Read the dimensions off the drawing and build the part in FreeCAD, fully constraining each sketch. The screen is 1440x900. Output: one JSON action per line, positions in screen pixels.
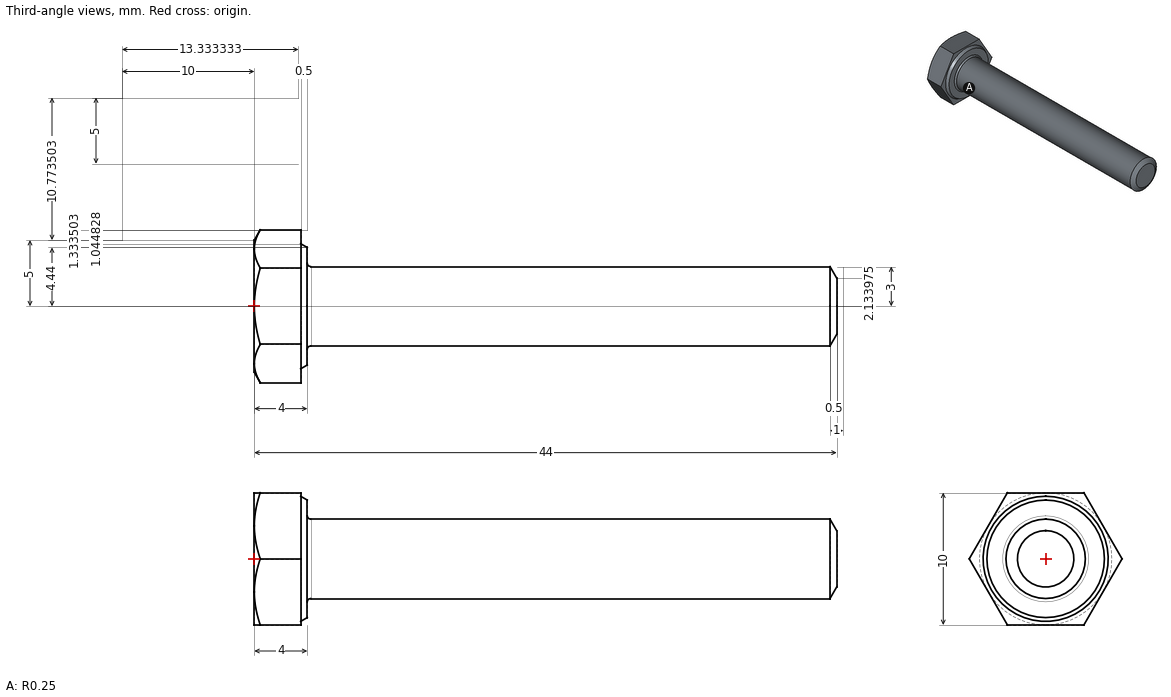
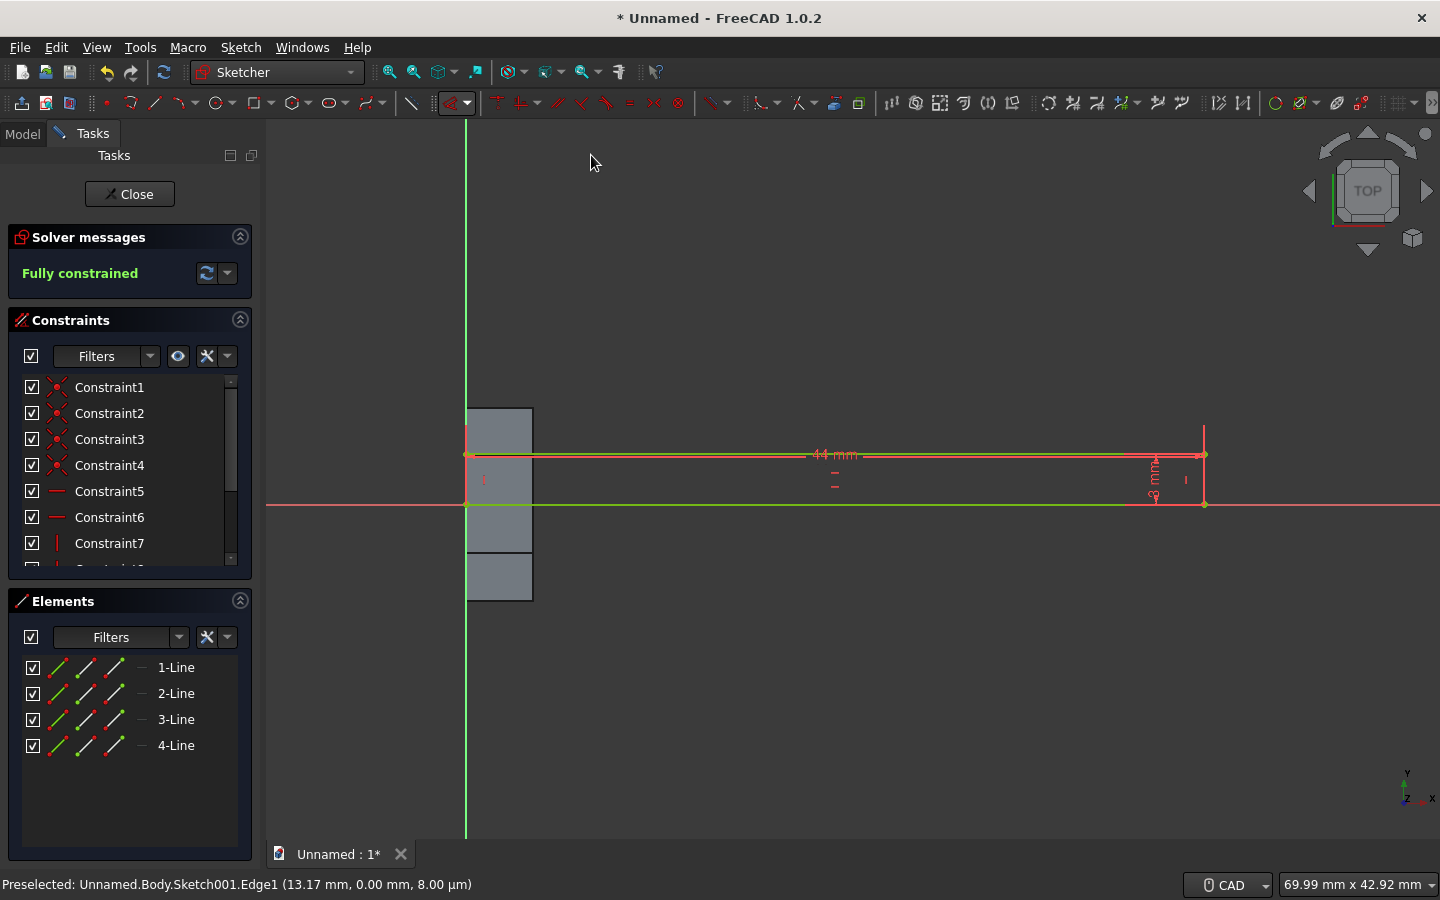
{"action": "left_click", "coordinate": [130, 194]}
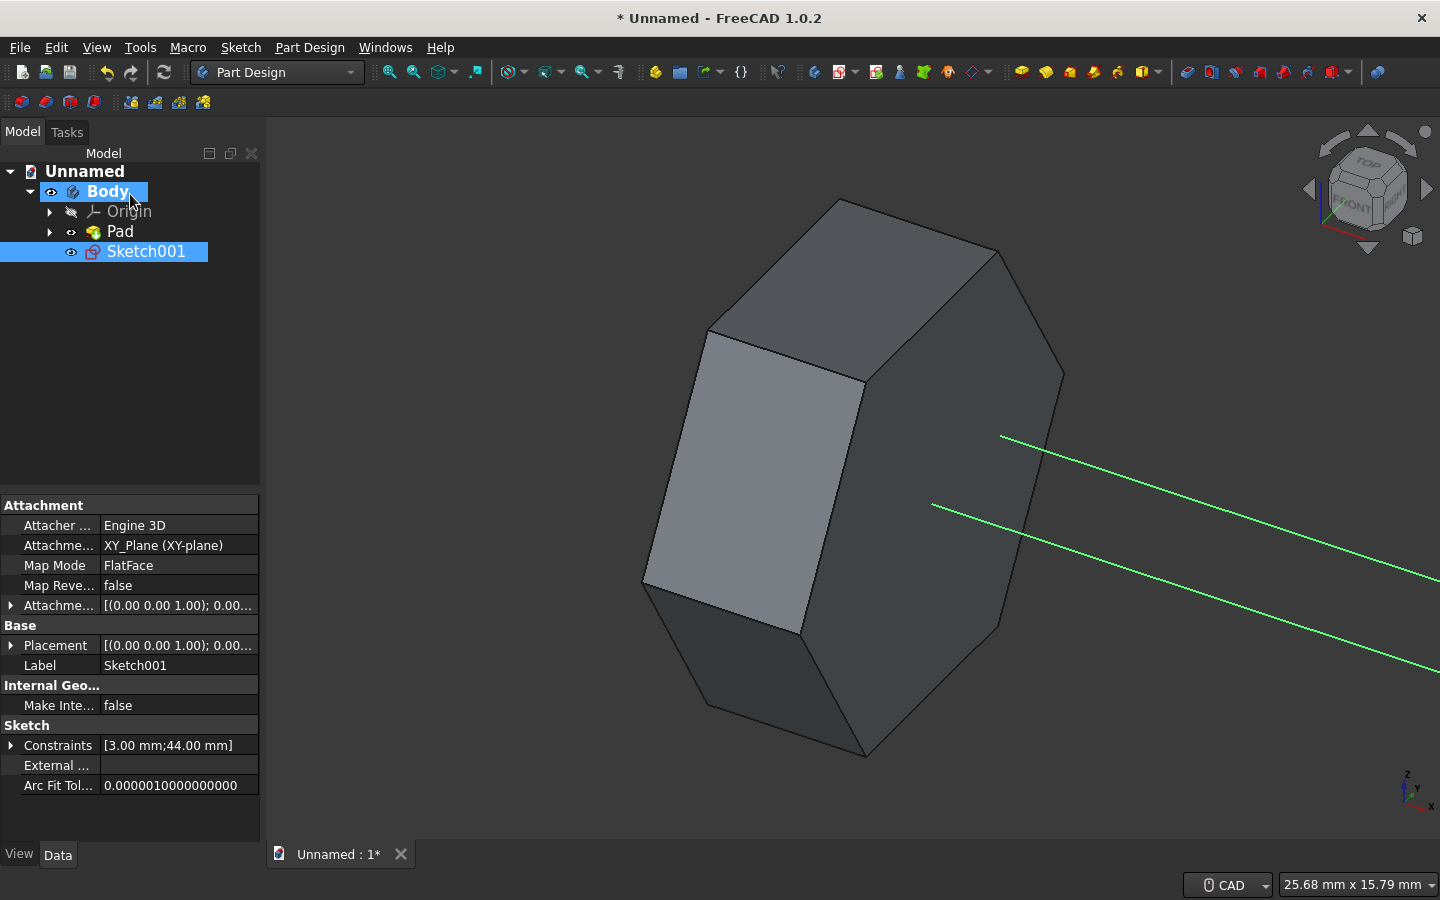
{"action": "left_click", "coordinate": [1046, 72]}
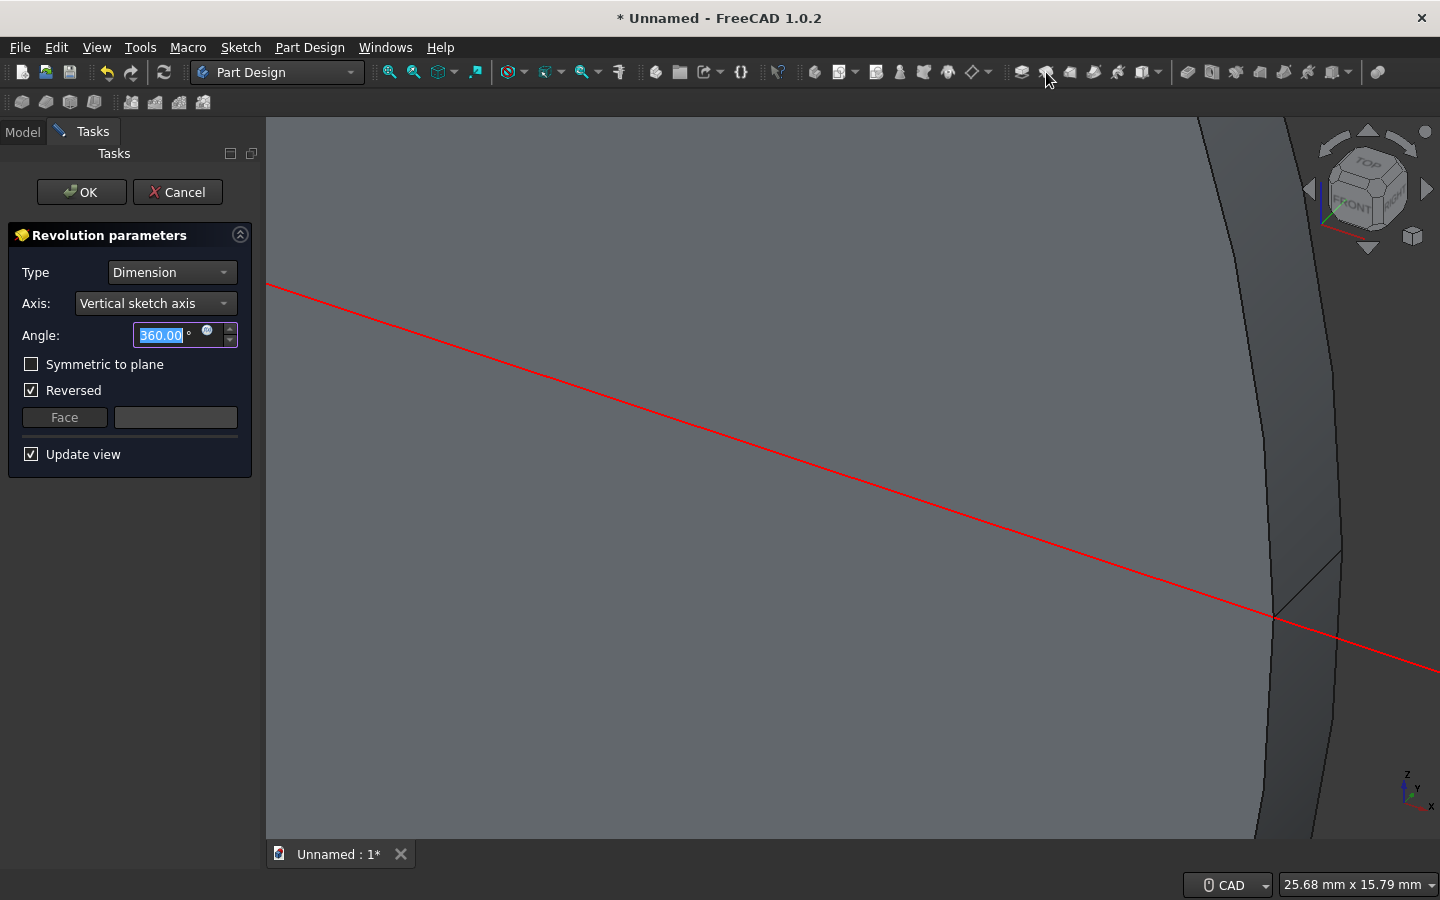
{"action": "left_click", "coordinate": [156, 304]}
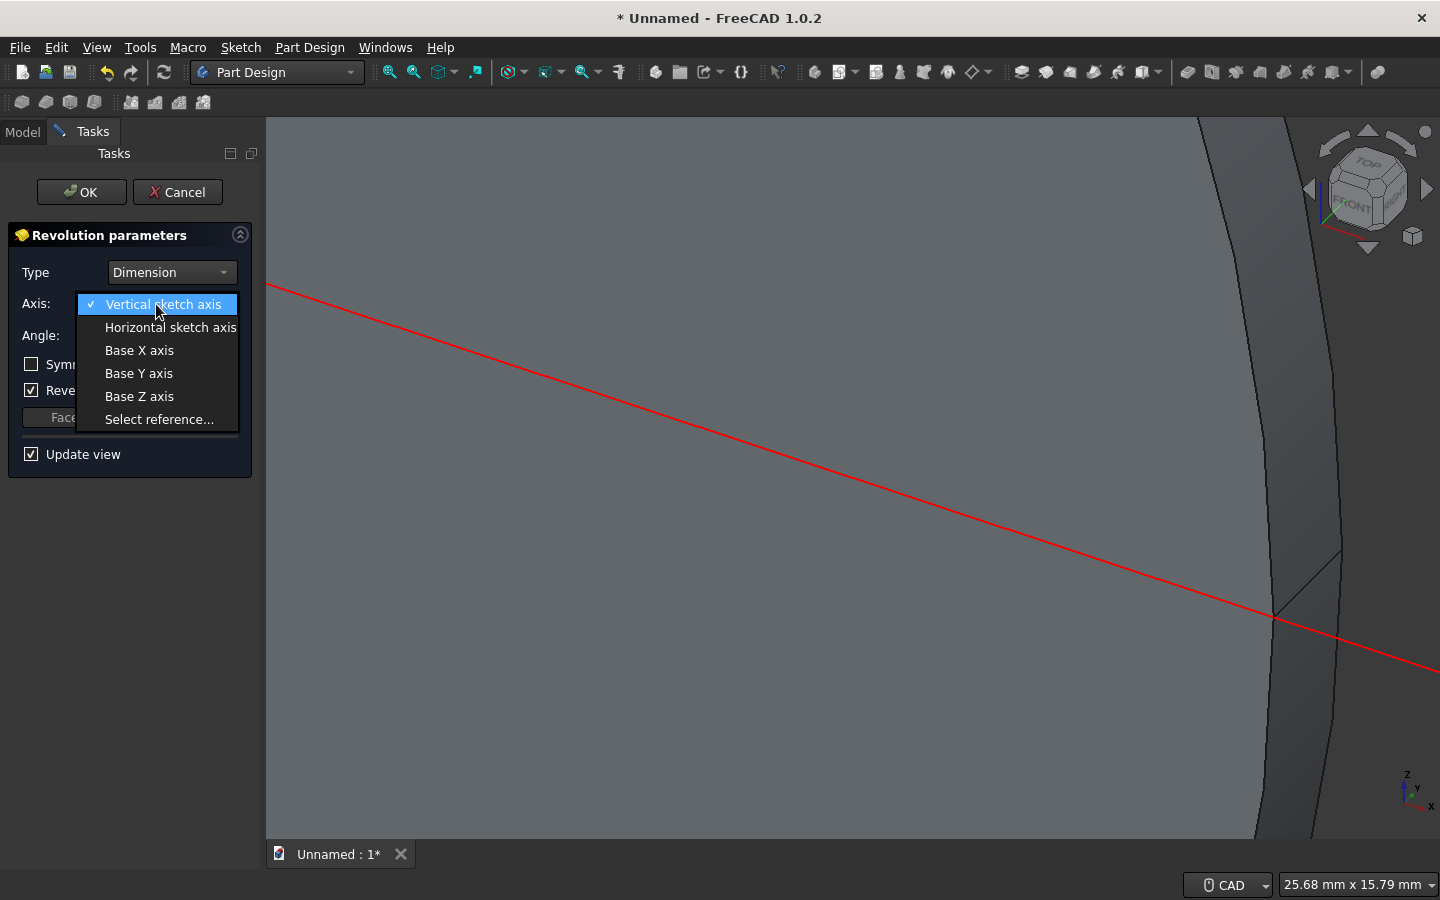
{"action": "left_click", "coordinate": [156, 328]}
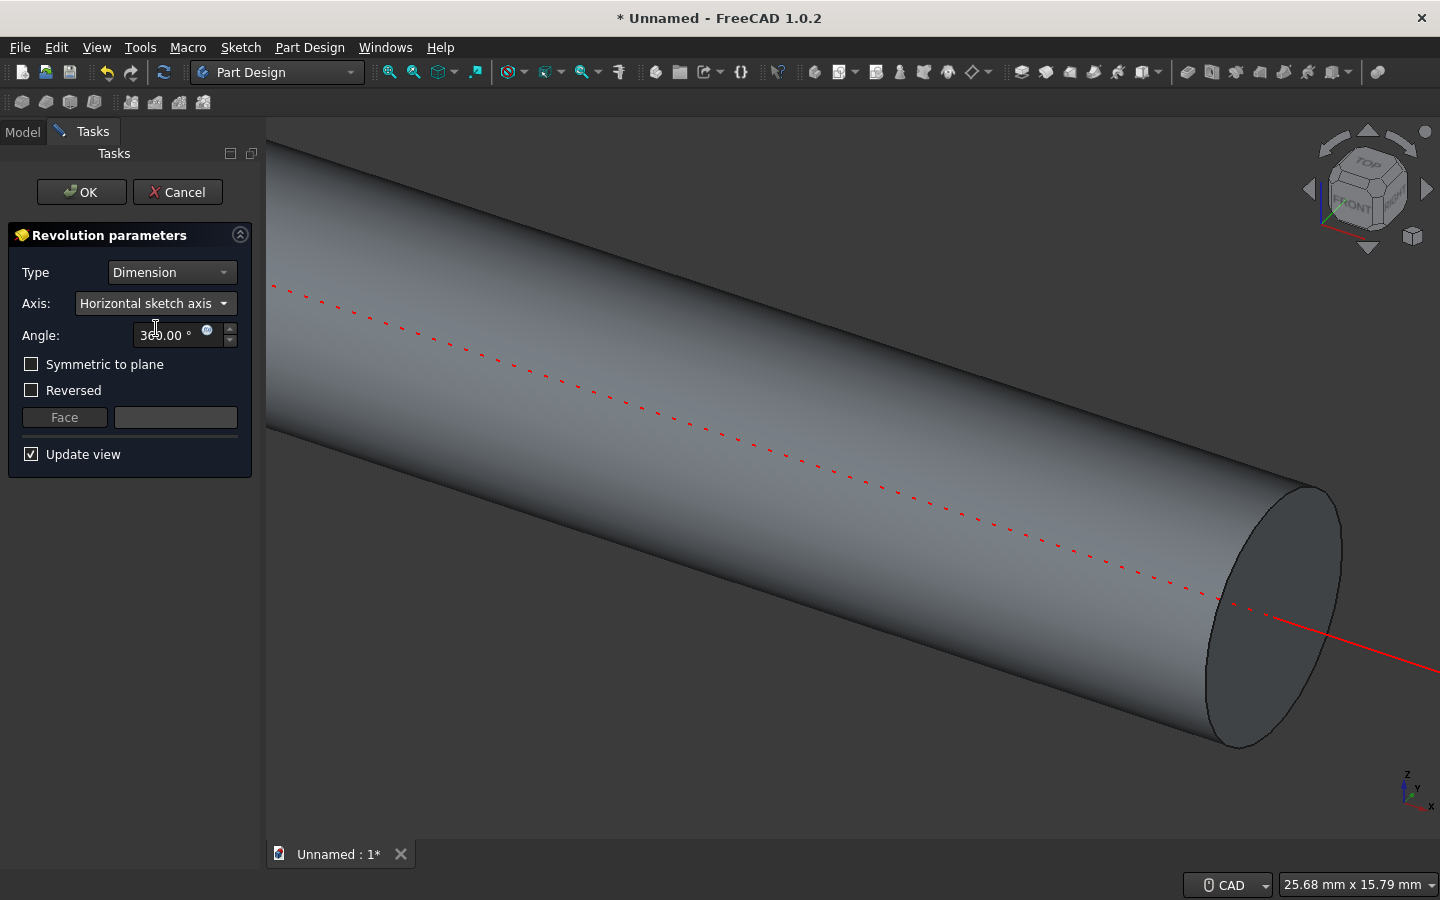
{"action": "left_click", "coordinate": [82, 192]}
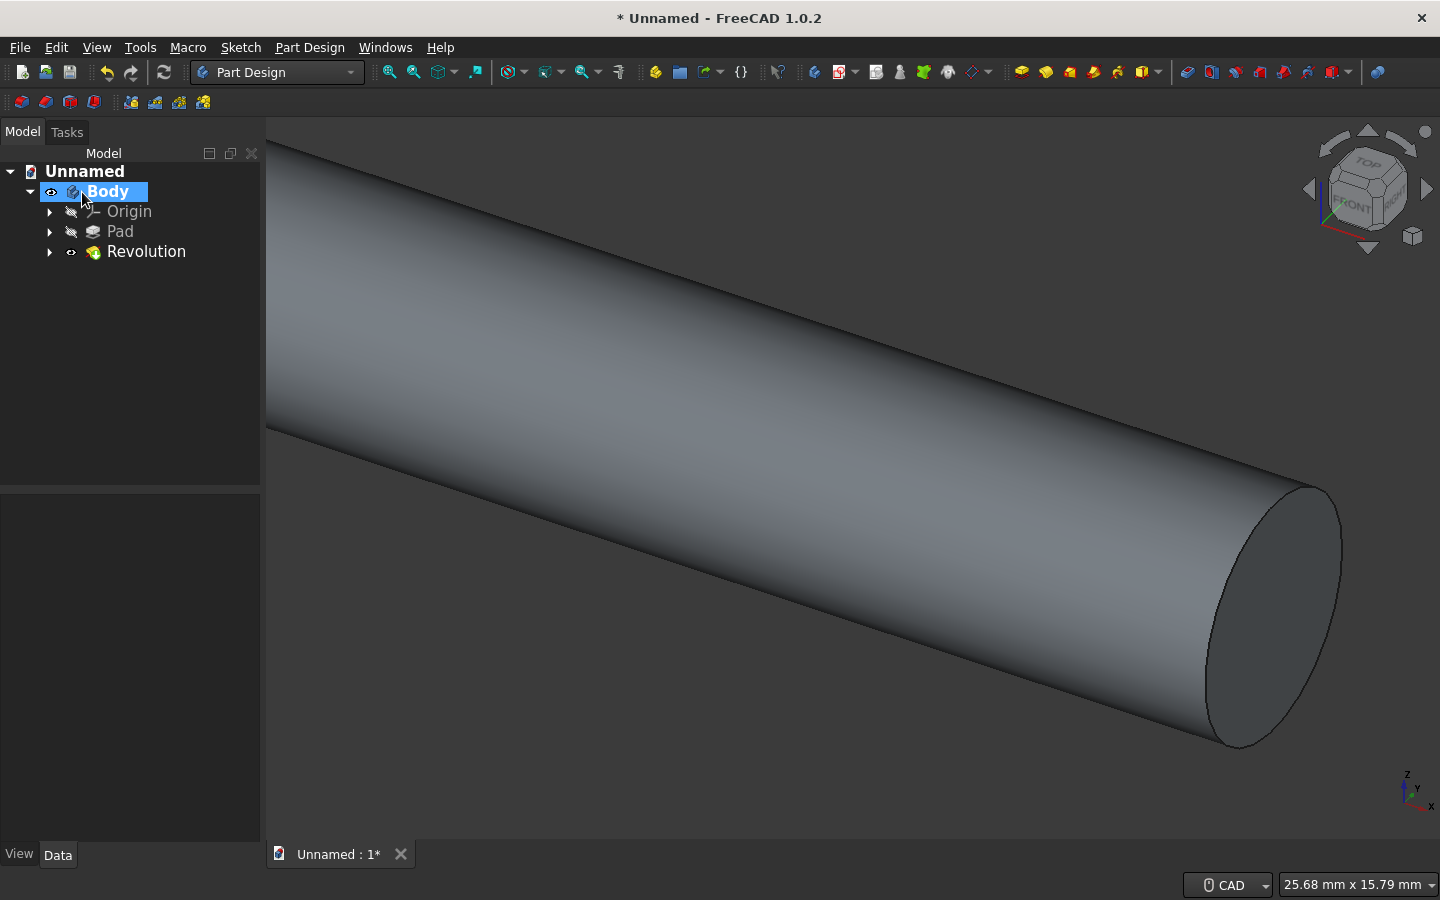
{"action": "left_click", "coordinate": [390, 72]}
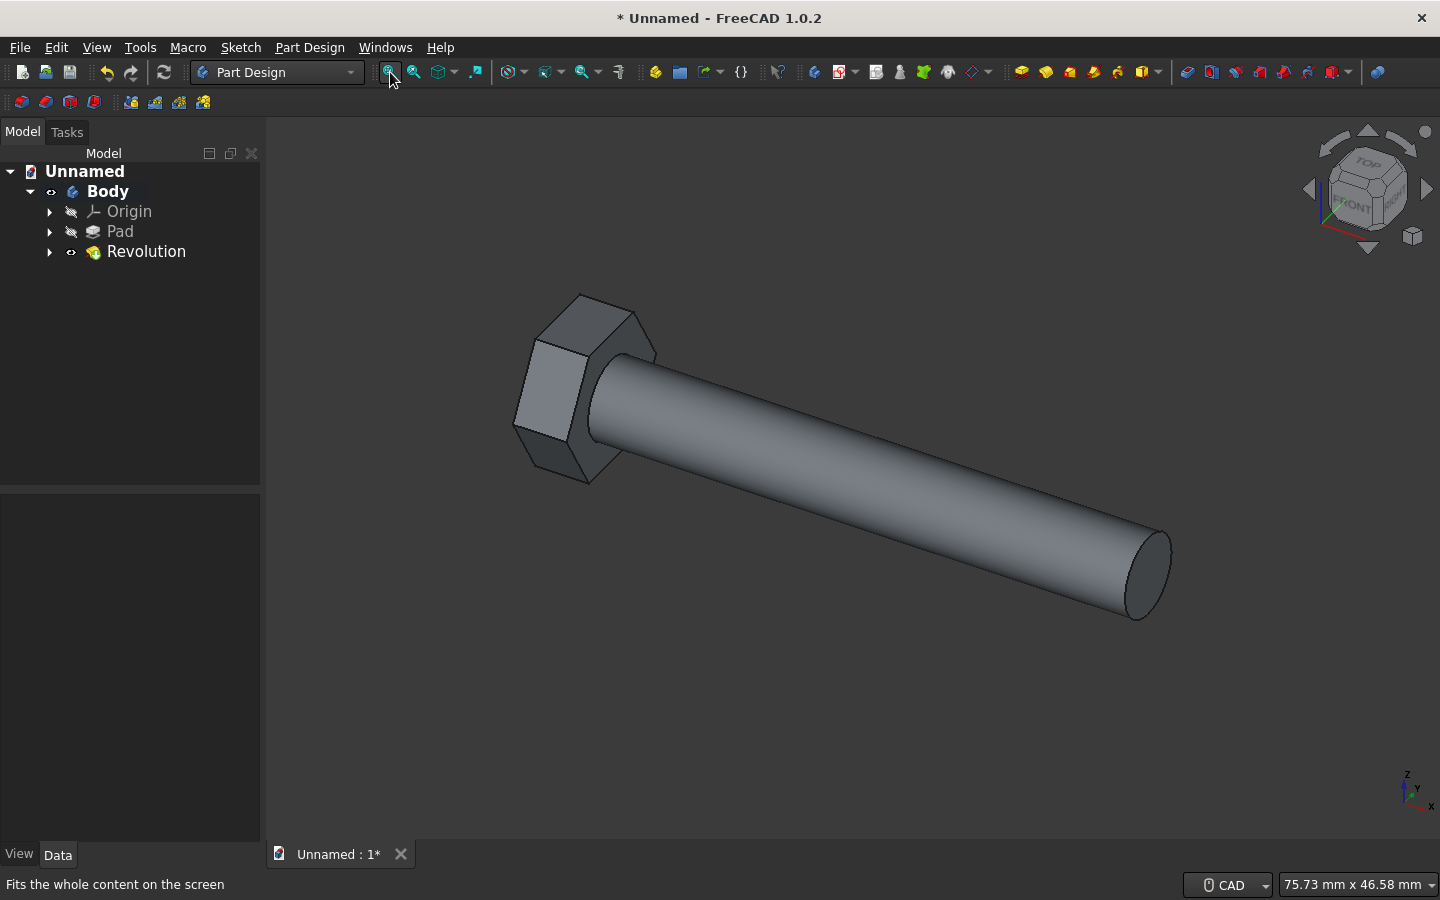
{"action": "left_click", "coordinate": [840, 72]}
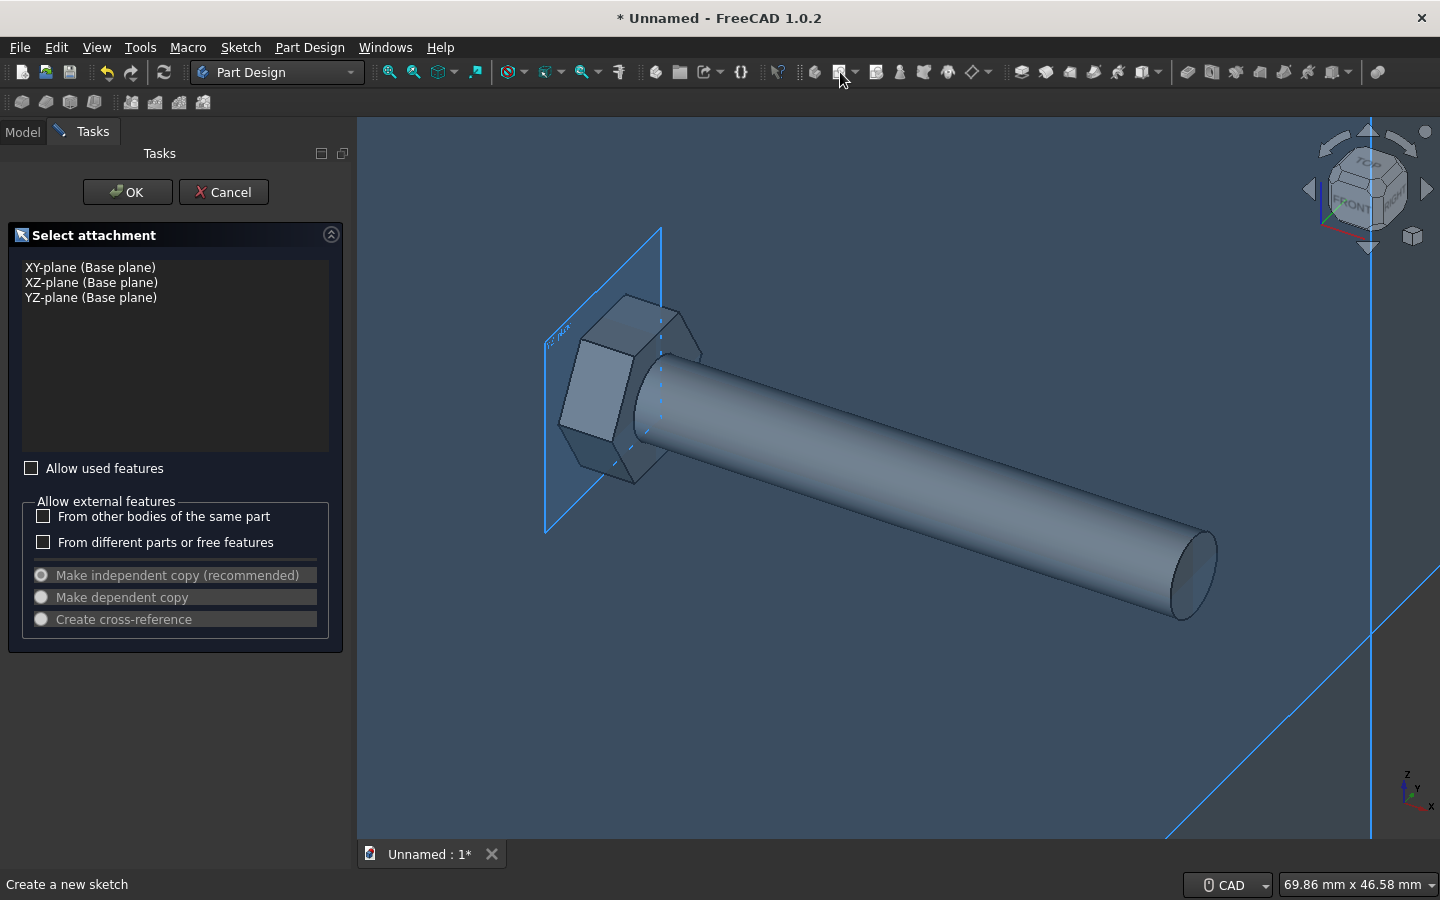
{"action": "left_click", "coordinate": [82, 268]}